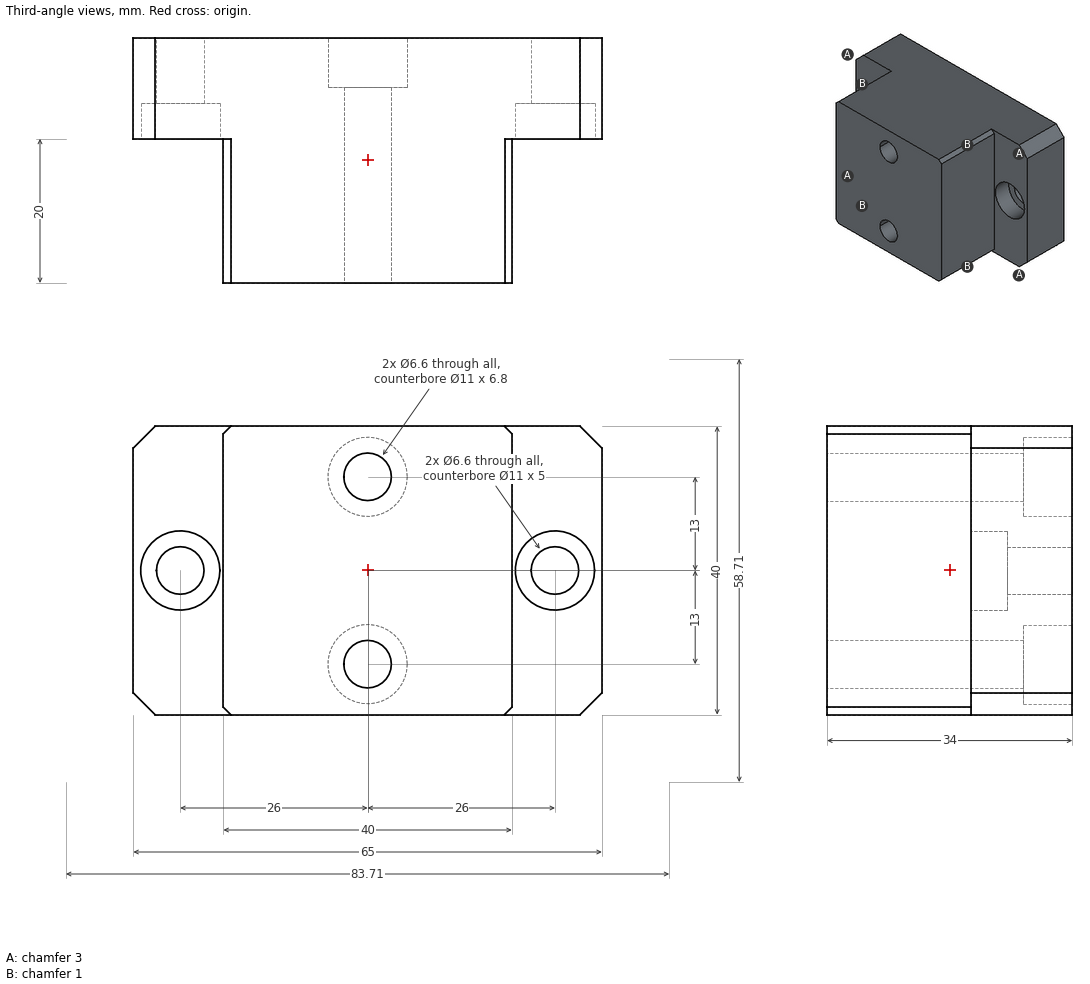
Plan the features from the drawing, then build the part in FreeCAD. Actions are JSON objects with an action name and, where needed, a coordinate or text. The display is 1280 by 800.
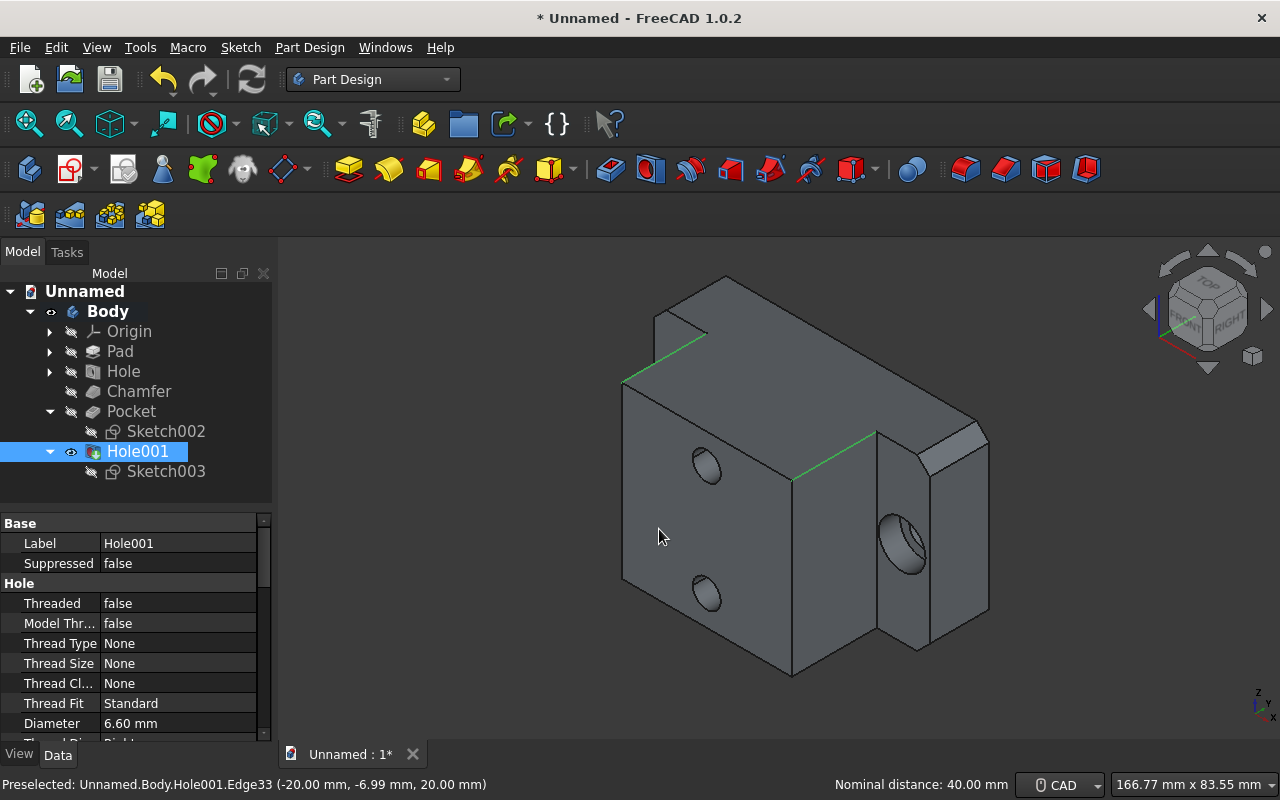
{"action": "key", "text": "1"}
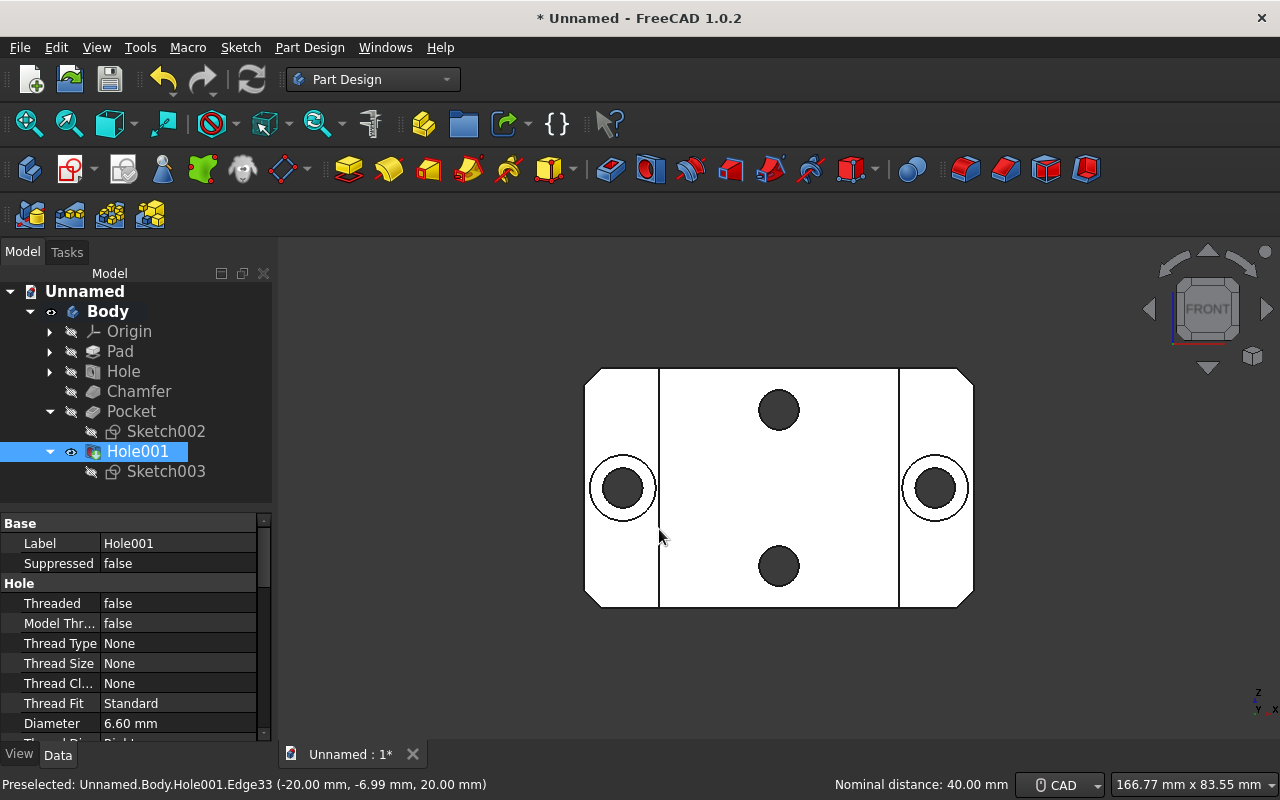
{"action": "key", "text": "3"}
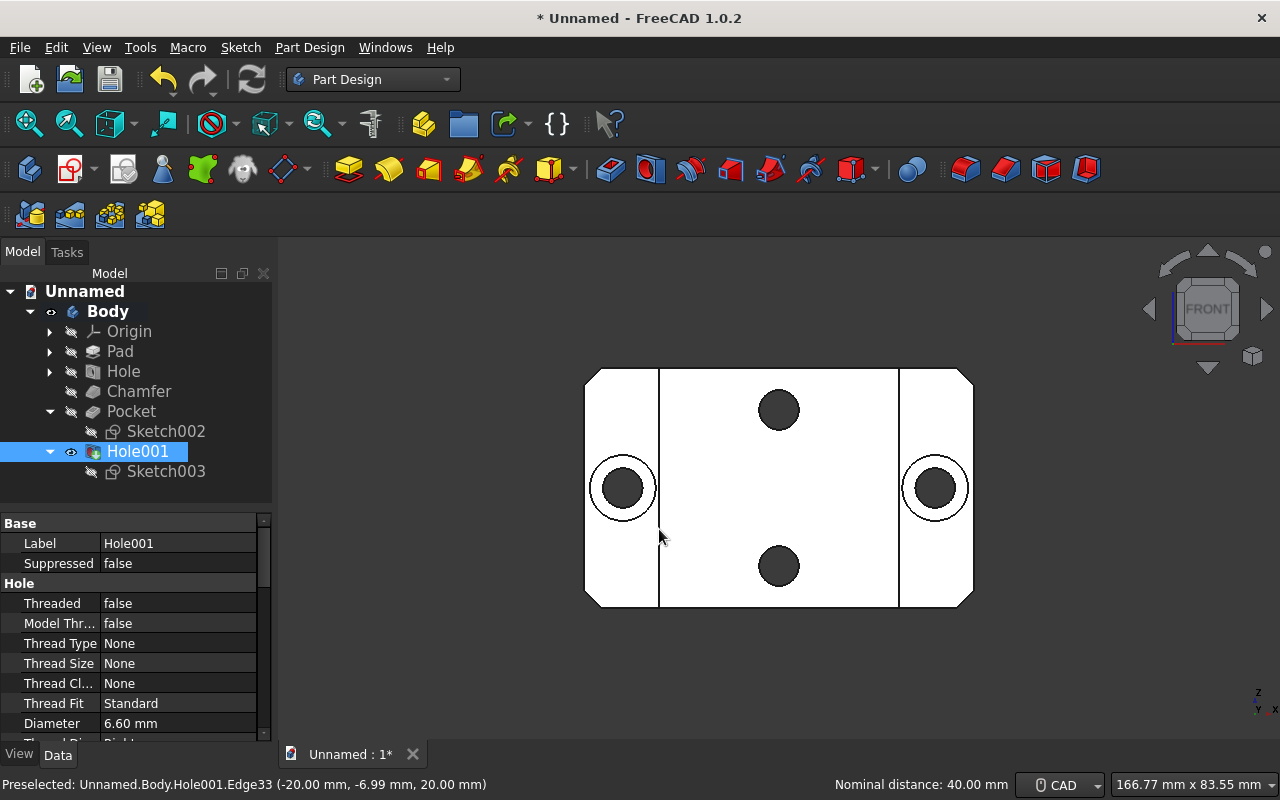
{"action": "left_click", "coordinate": [737, 607], "text": "ctrl"}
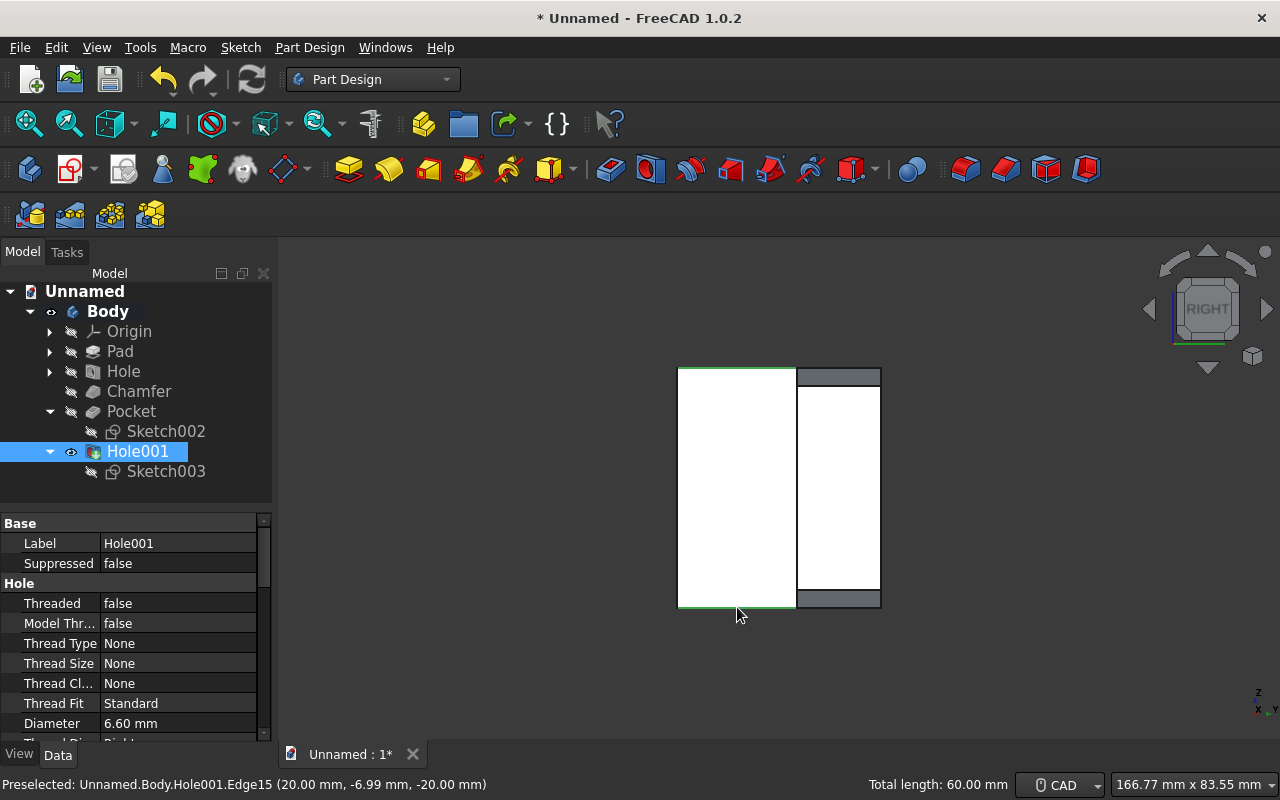
{"action": "key", "text": "5"}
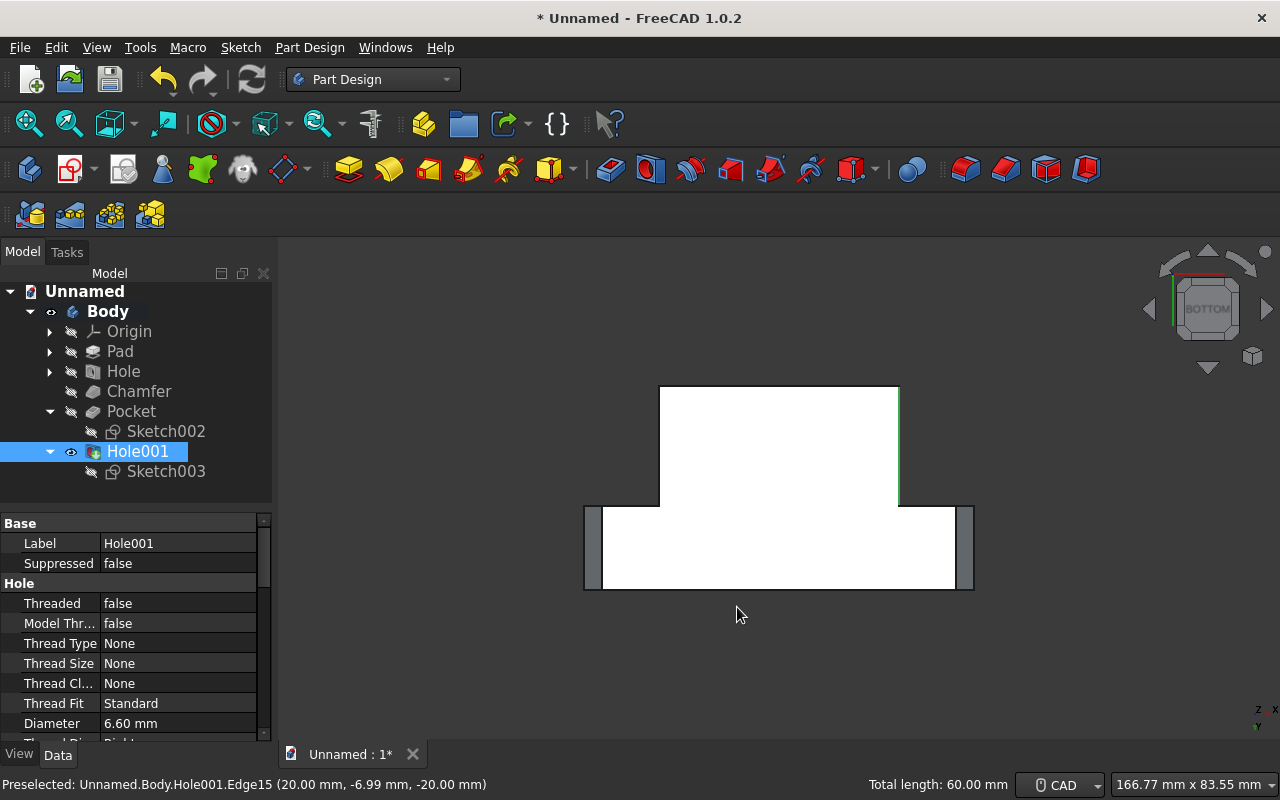
{"action": "left_click", "coordinate": [30, 124]}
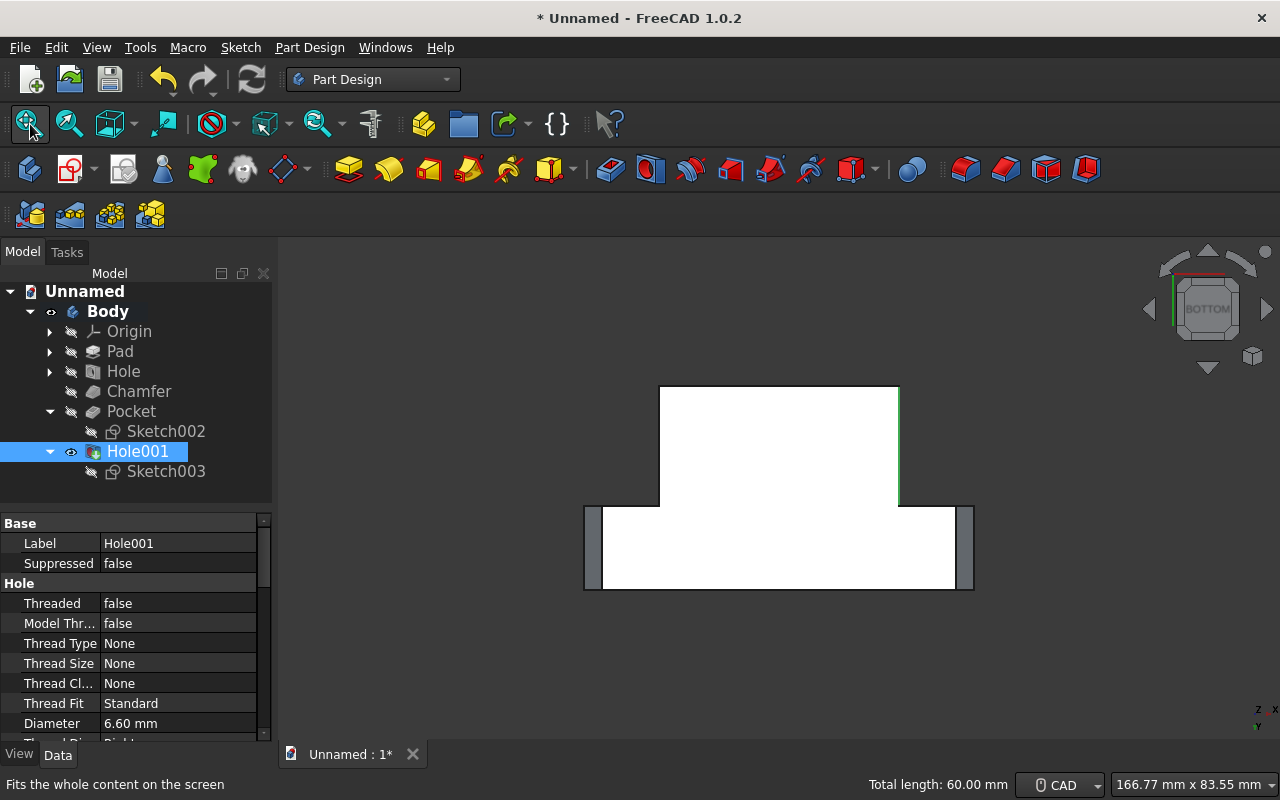
{"action": "left_click", "coordinate": [659, 445], "text": "ctrl"}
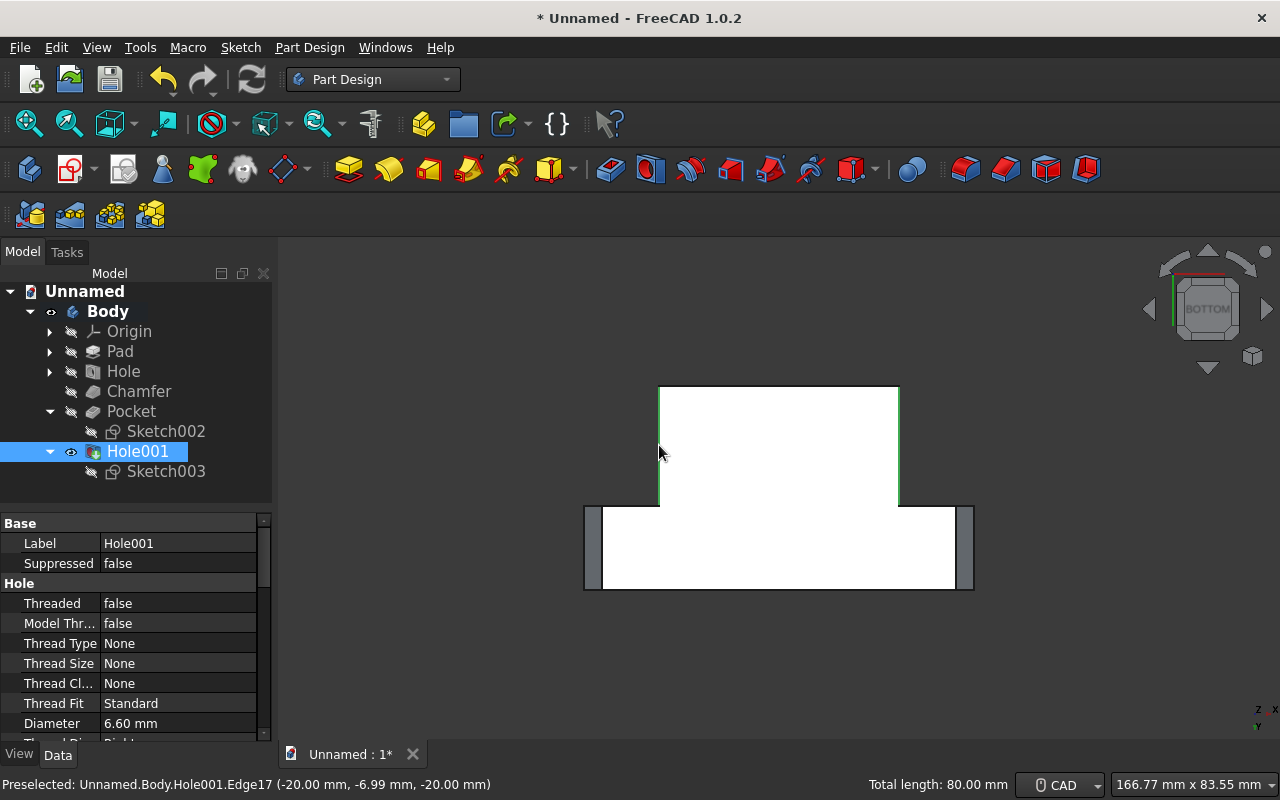
{"action": "left_click", "coordinate": [1006, 170]}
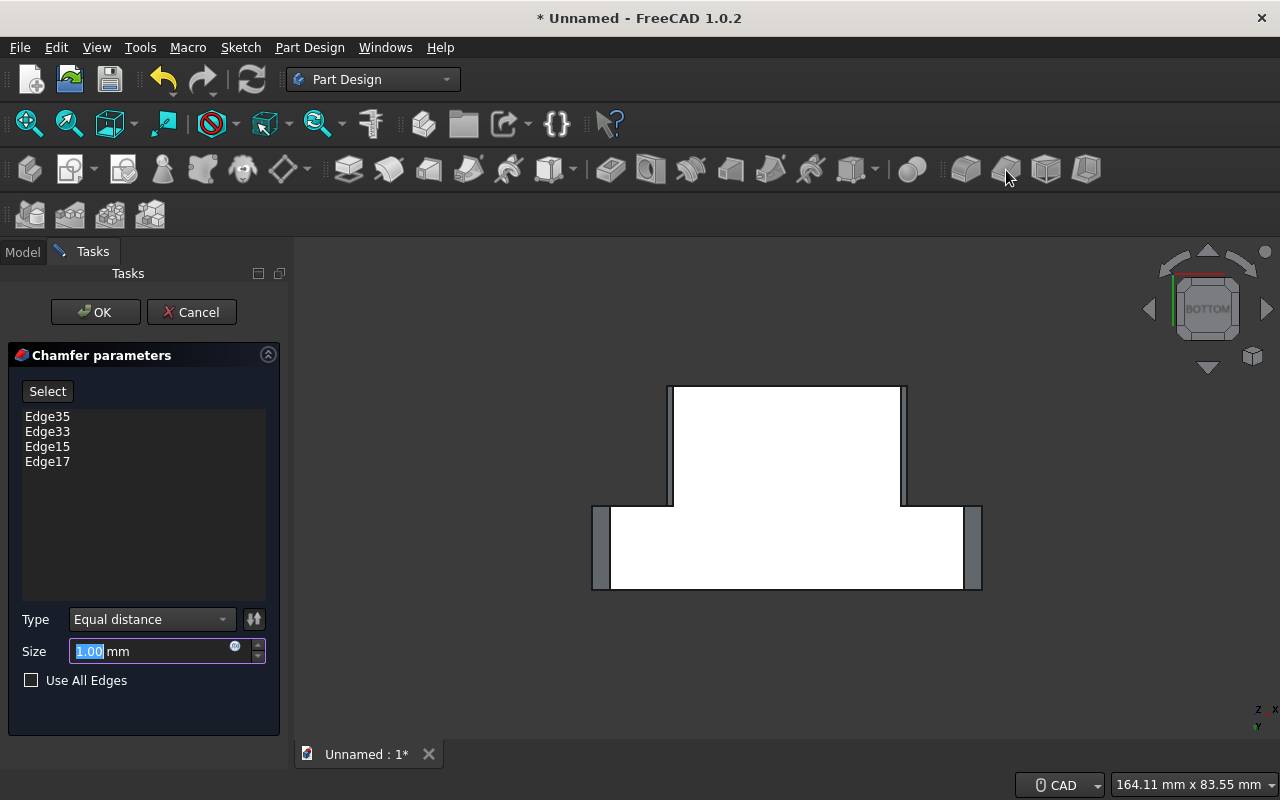
{"action": "type", "text": "1"}
{"action": "key", "text": "Tab"}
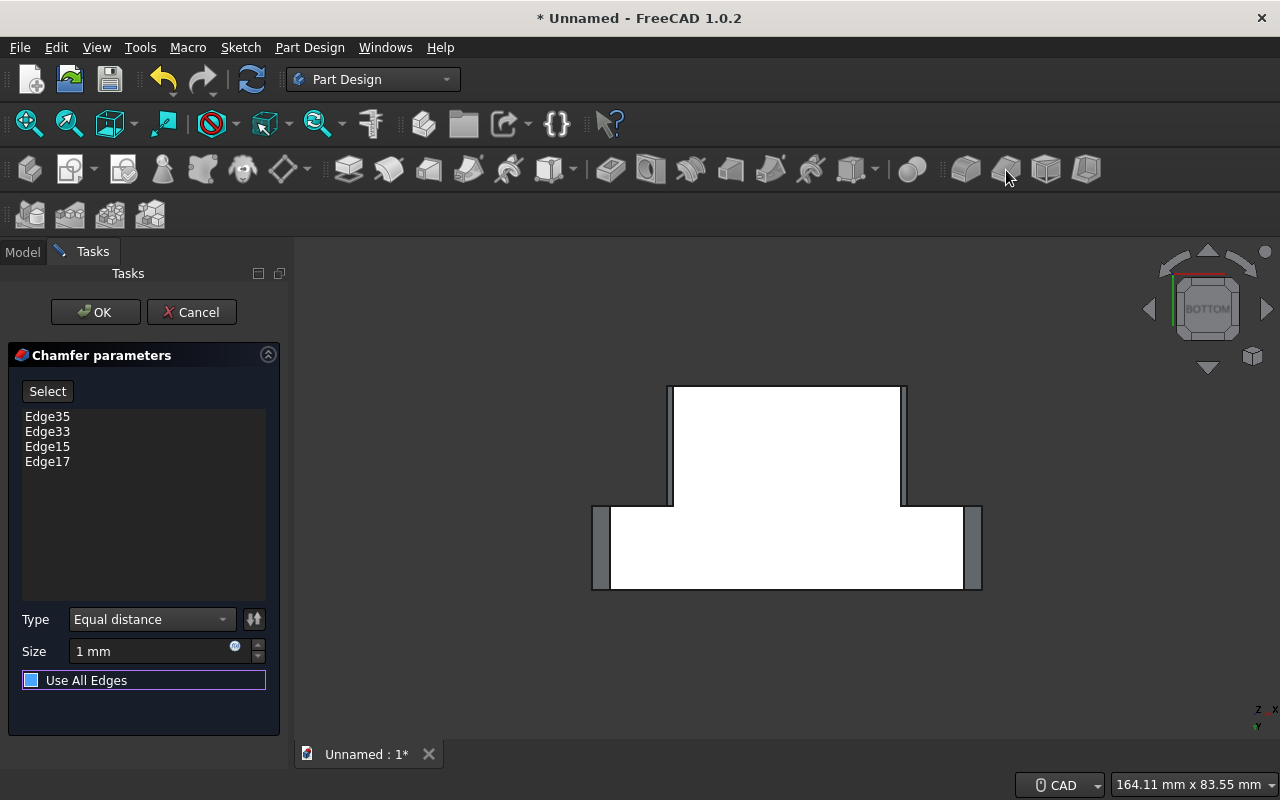
{"action": "left_click", "coordinate": [96, 312]}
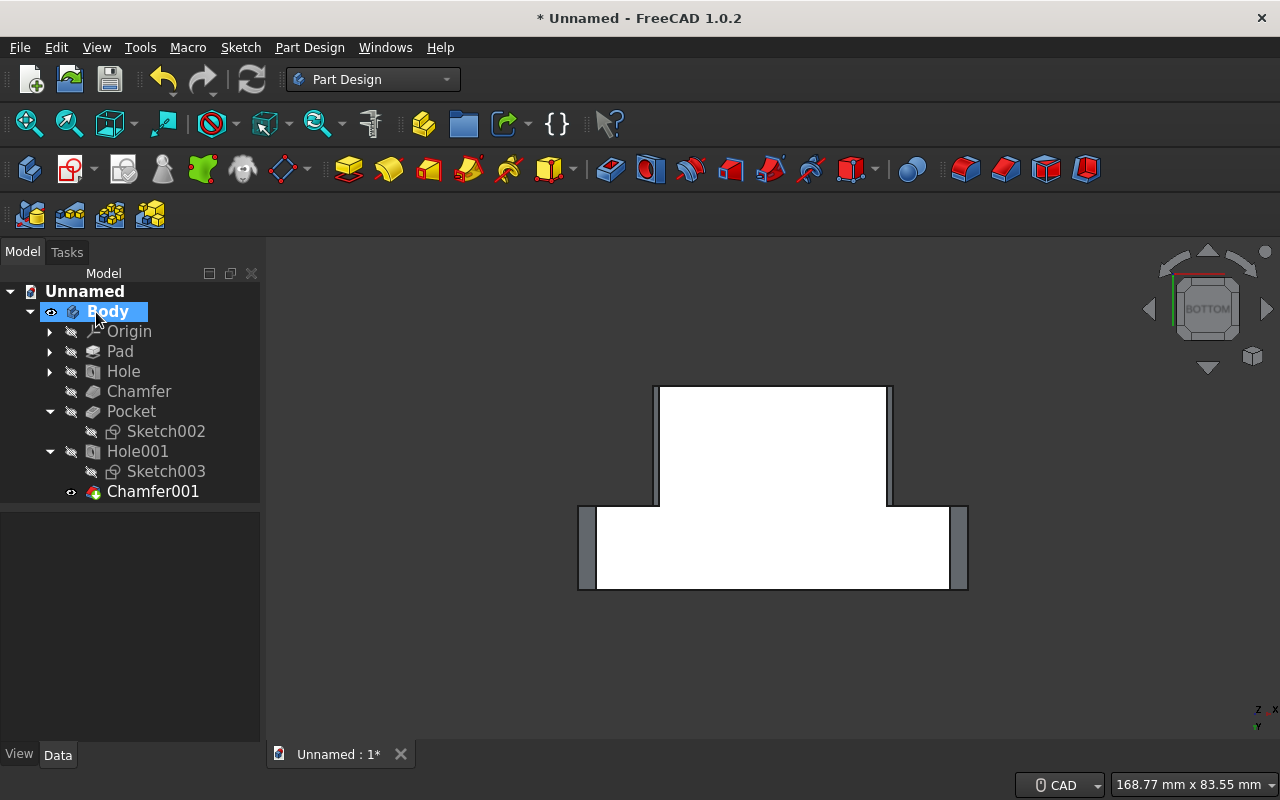
{"action": "key", "text": "0"}